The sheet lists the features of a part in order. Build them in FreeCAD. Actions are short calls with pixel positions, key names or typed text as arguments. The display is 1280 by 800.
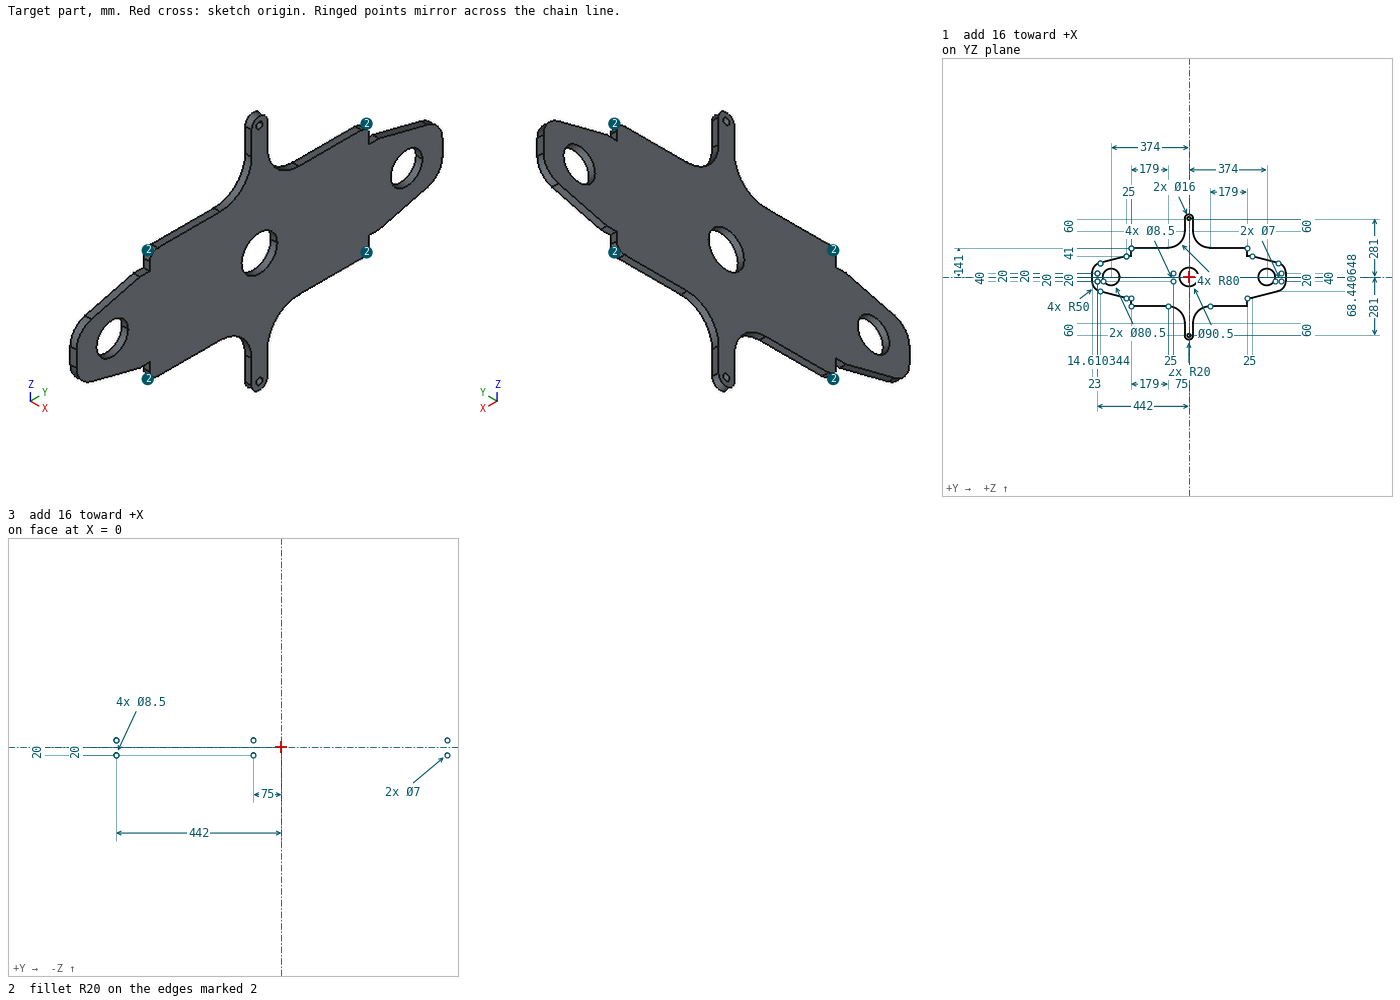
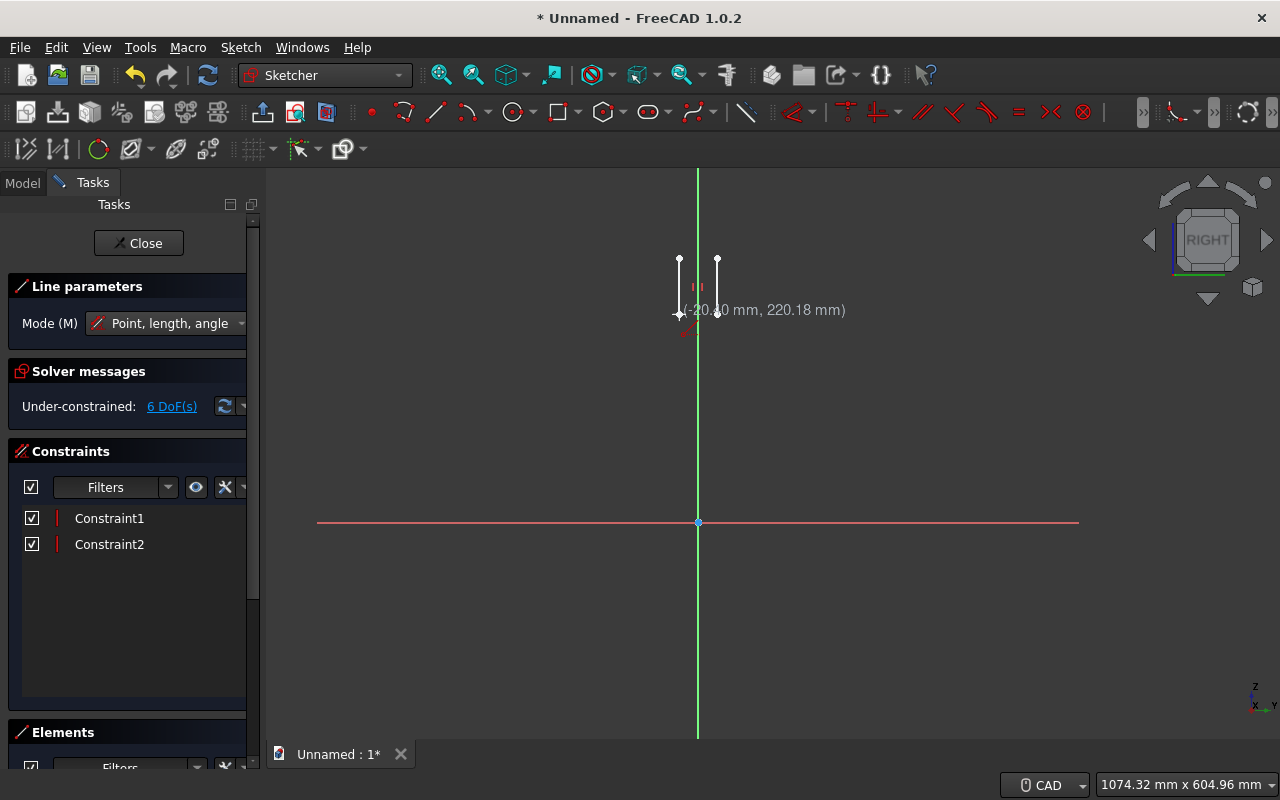
click(404, 112)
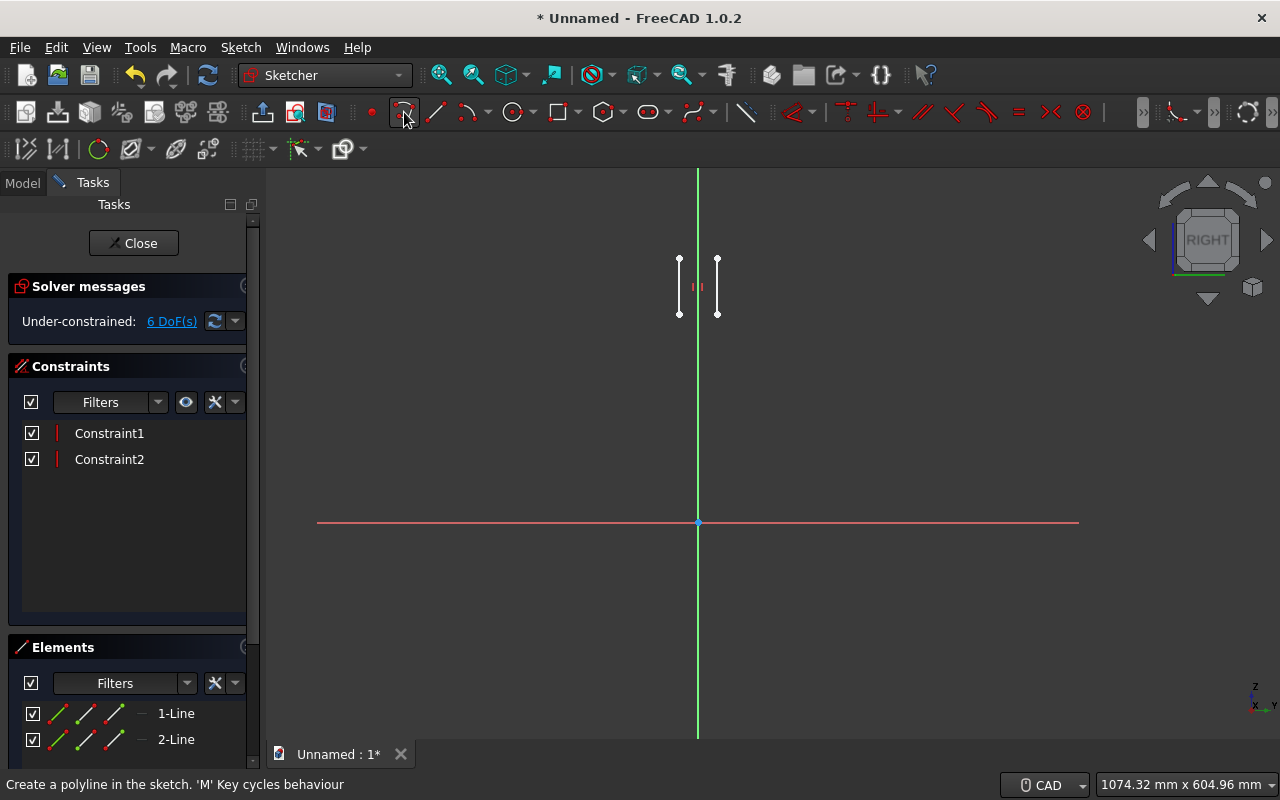
click(604, 390)
click(435, 390)
click(435, 428)
click(411, 428)
click(295, 458)
right_click(295, 458)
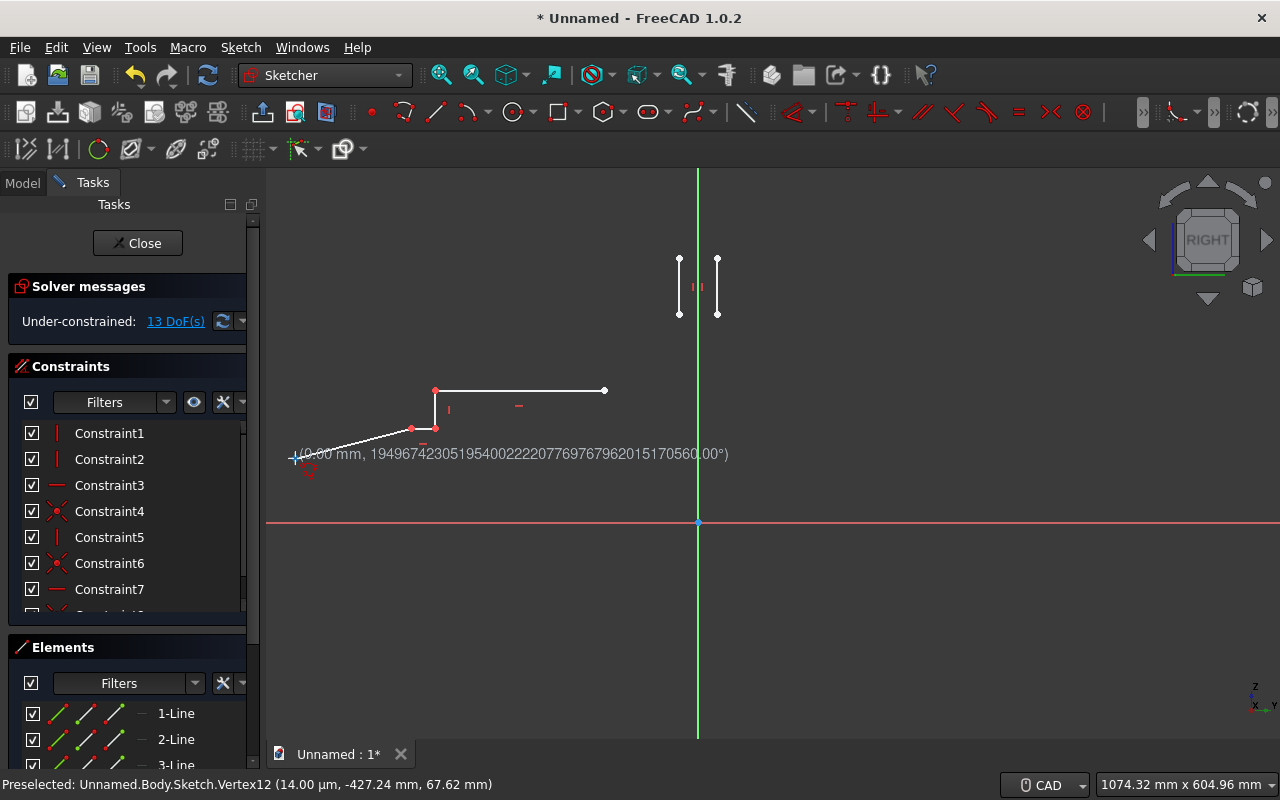
click(436, 112)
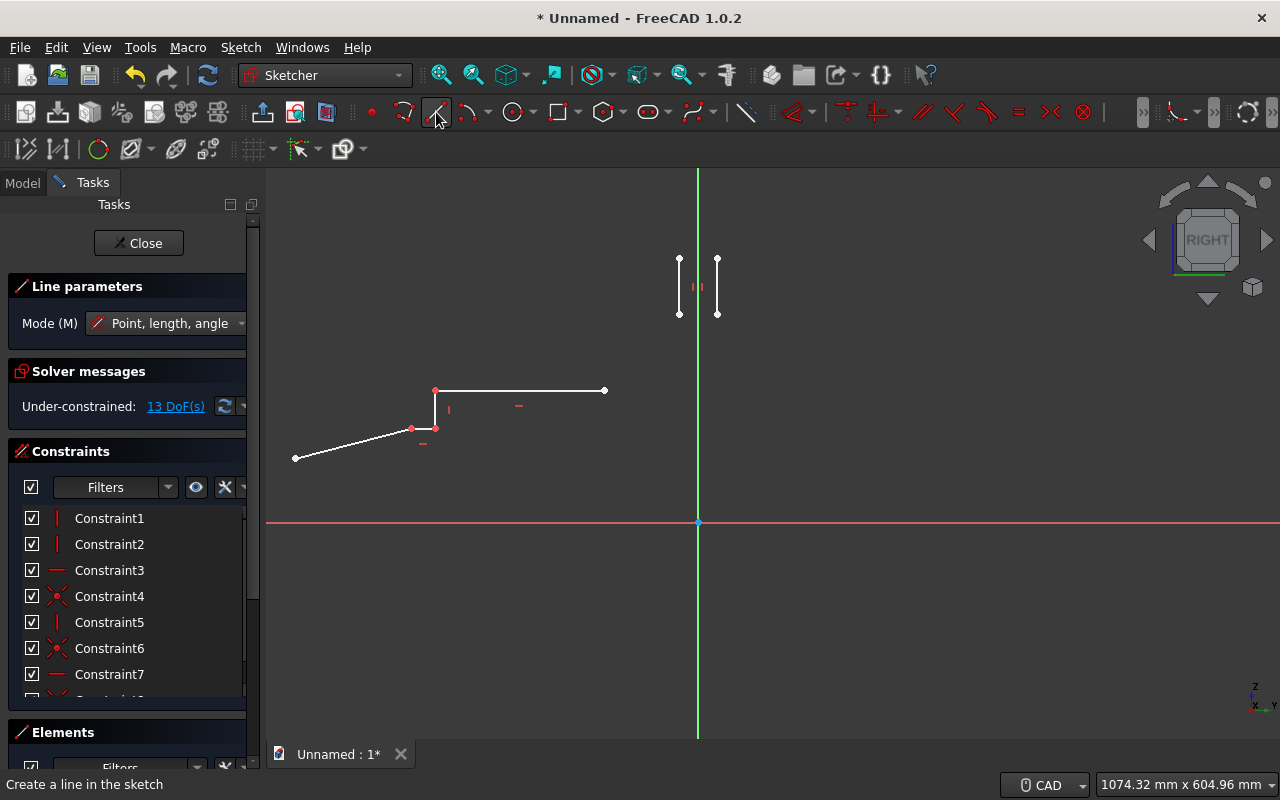
scroll(717, 313, down, 2)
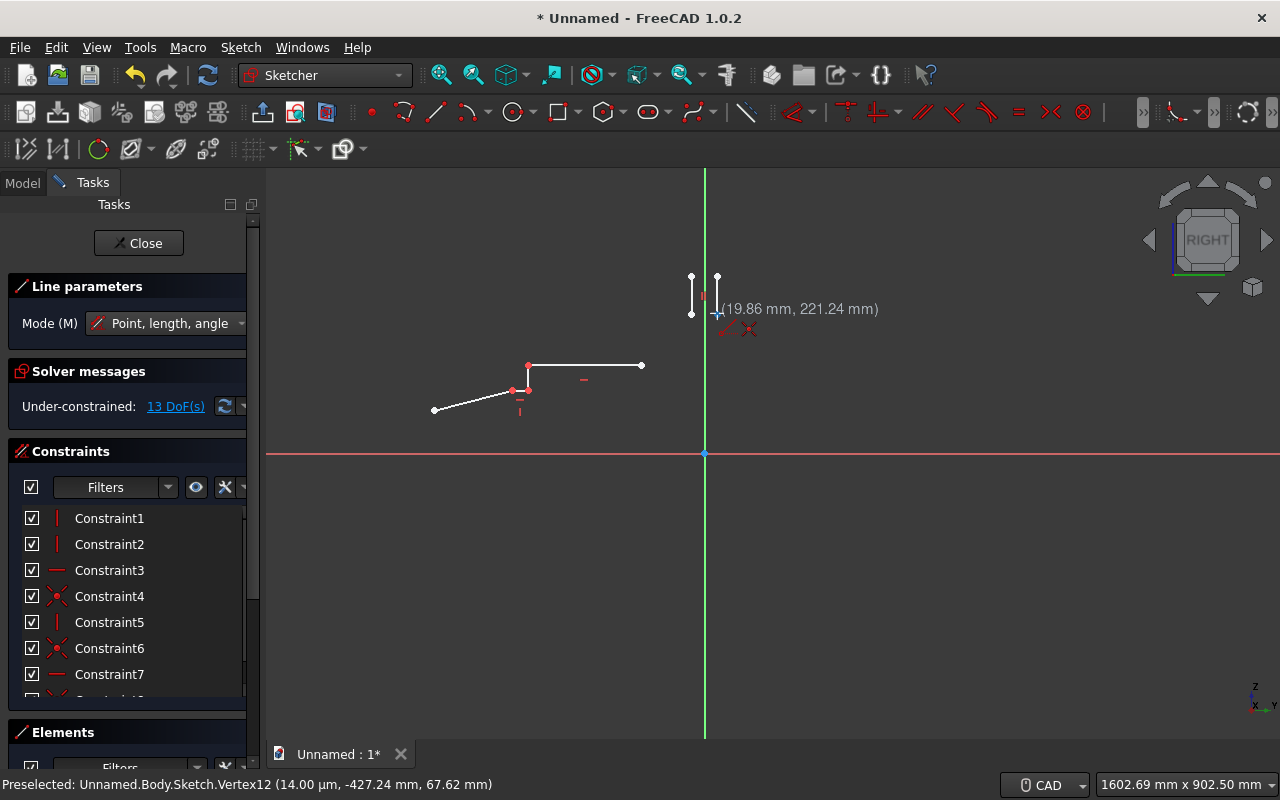
scroll(410, 441, up, 2)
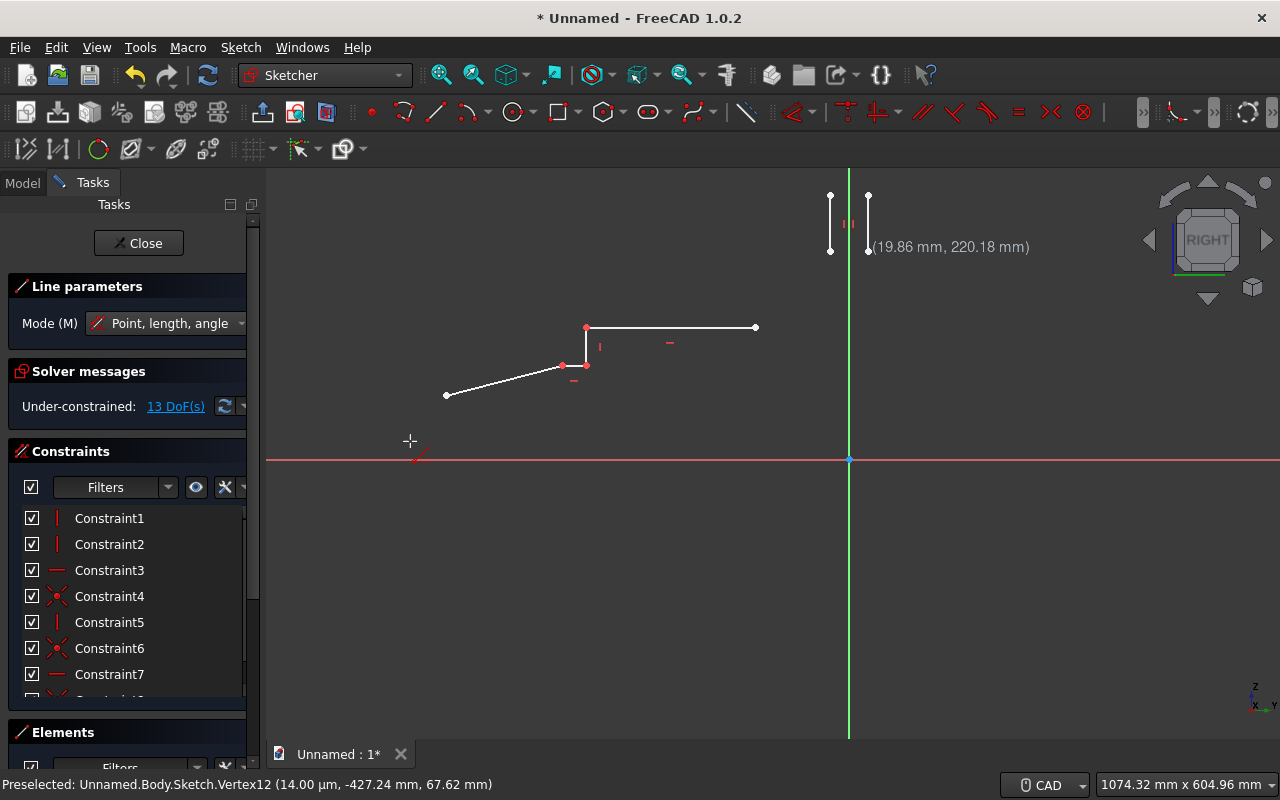
click(410, 441)
click(410, 479)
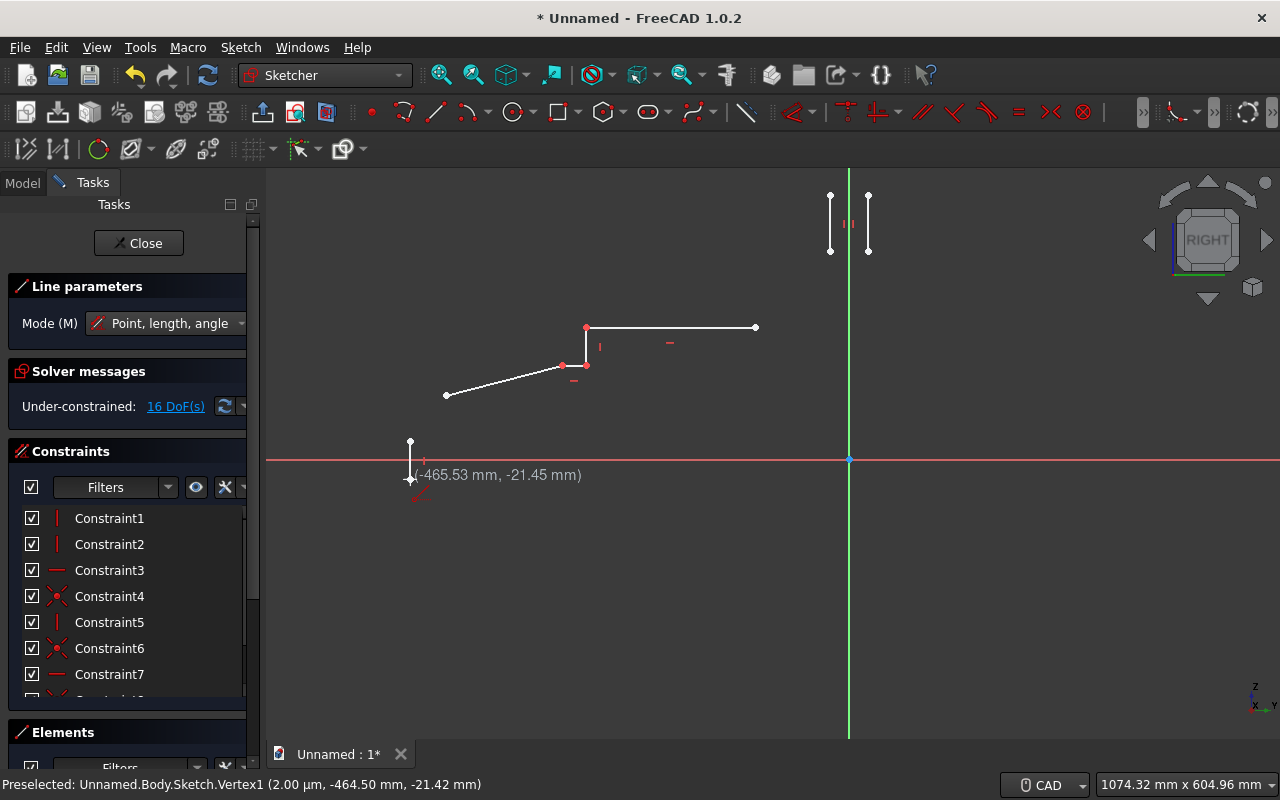
click(404, 112)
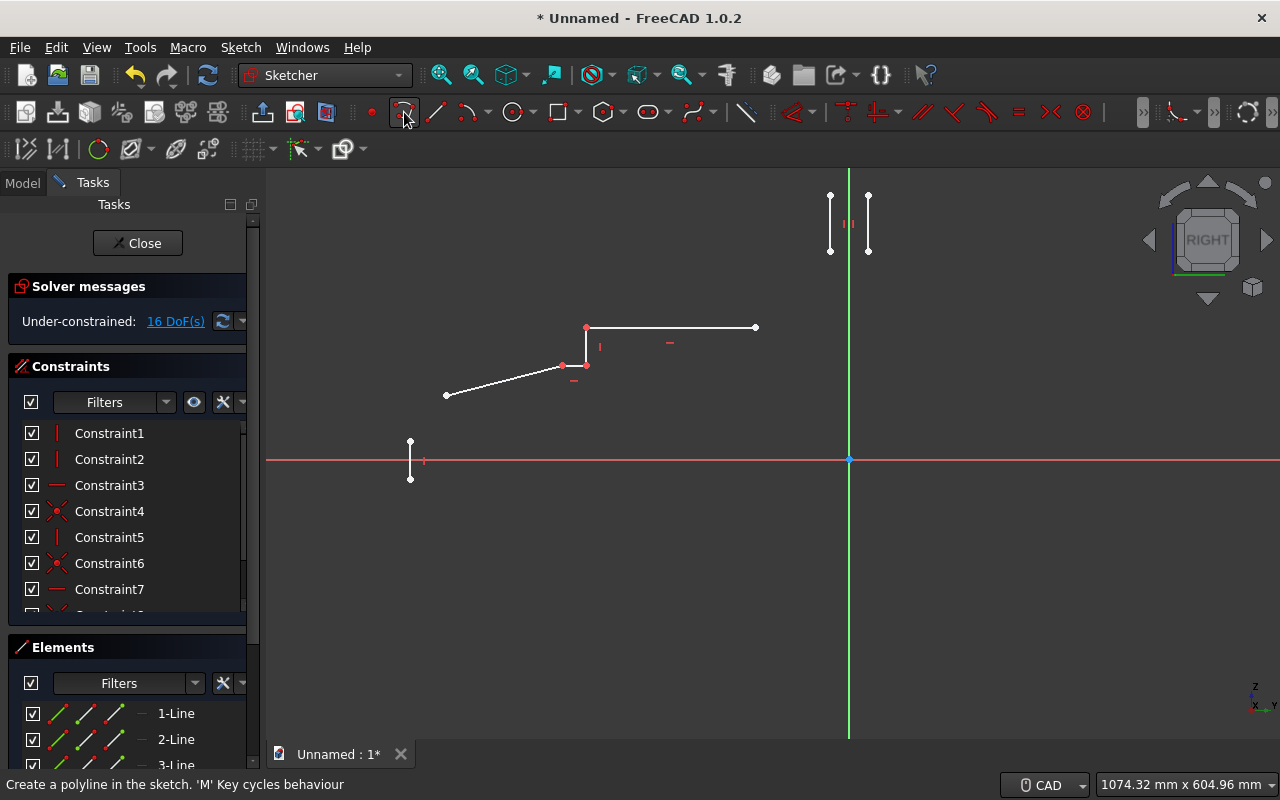
click(446, 524)
click(562, 554)
click(586, 554)
click(586, 593)
click(755, 593)
right_click(755, 593)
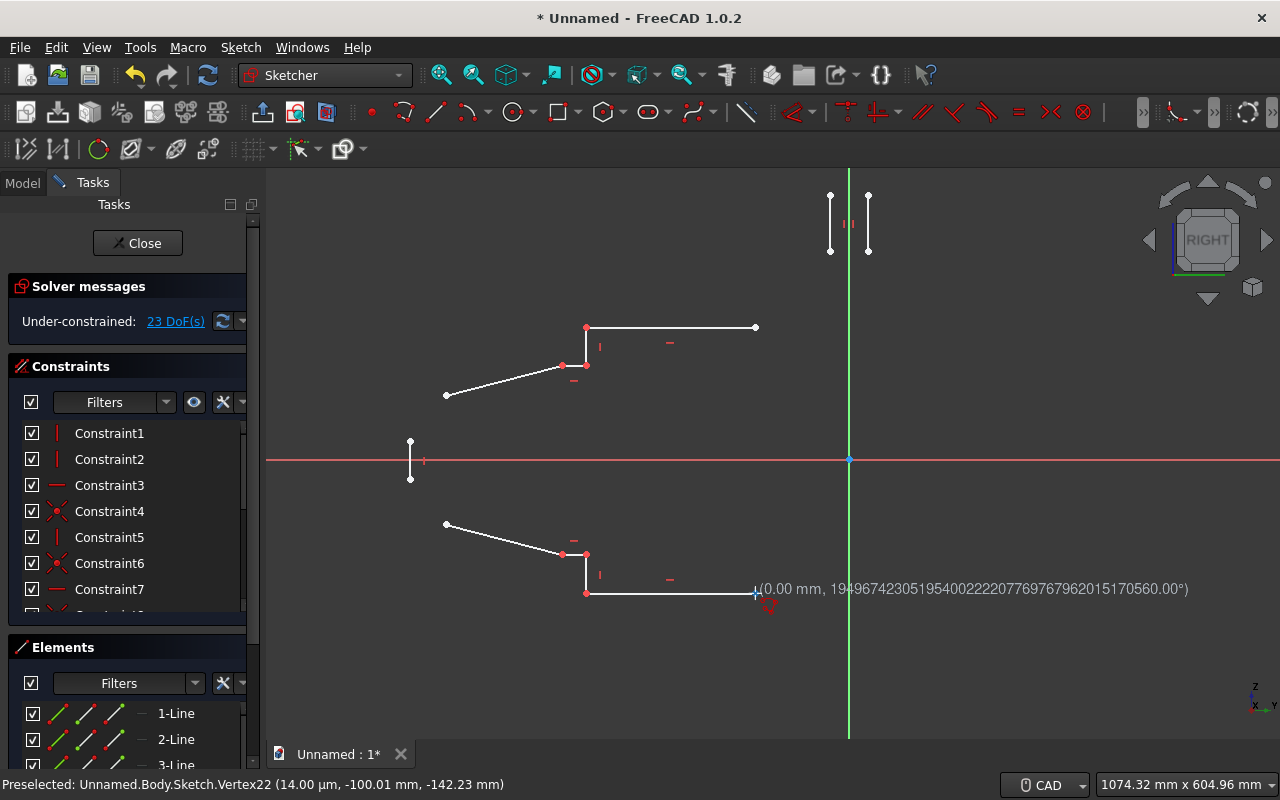
click(436, 112)